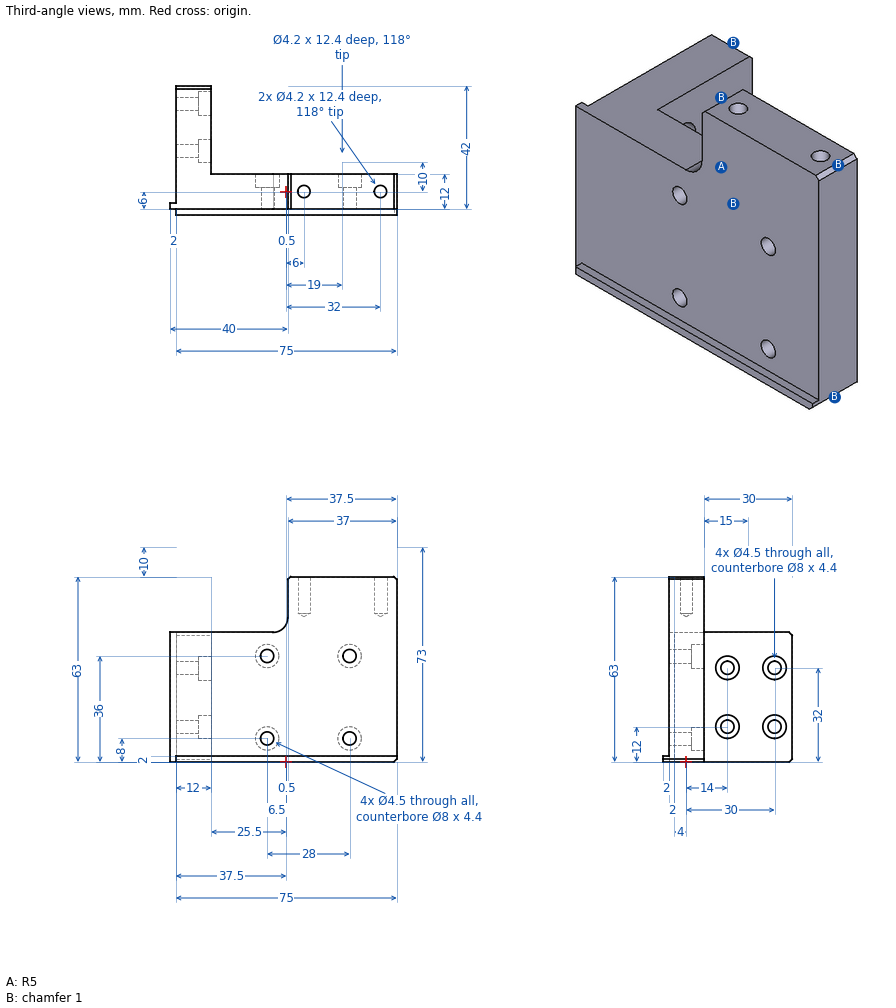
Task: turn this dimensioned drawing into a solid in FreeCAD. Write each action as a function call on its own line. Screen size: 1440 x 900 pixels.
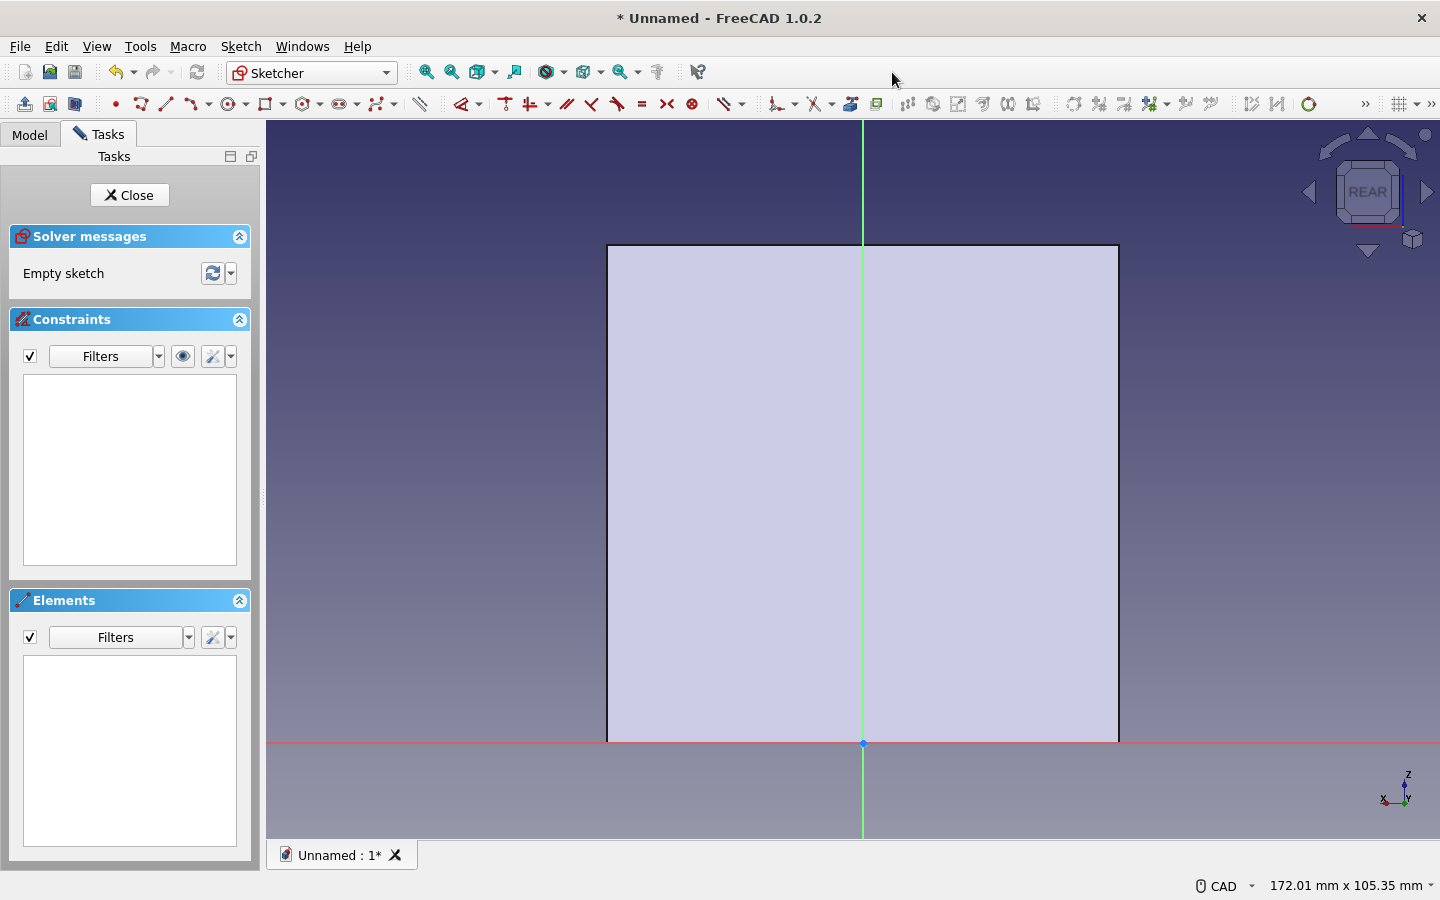
key(g)
key(r)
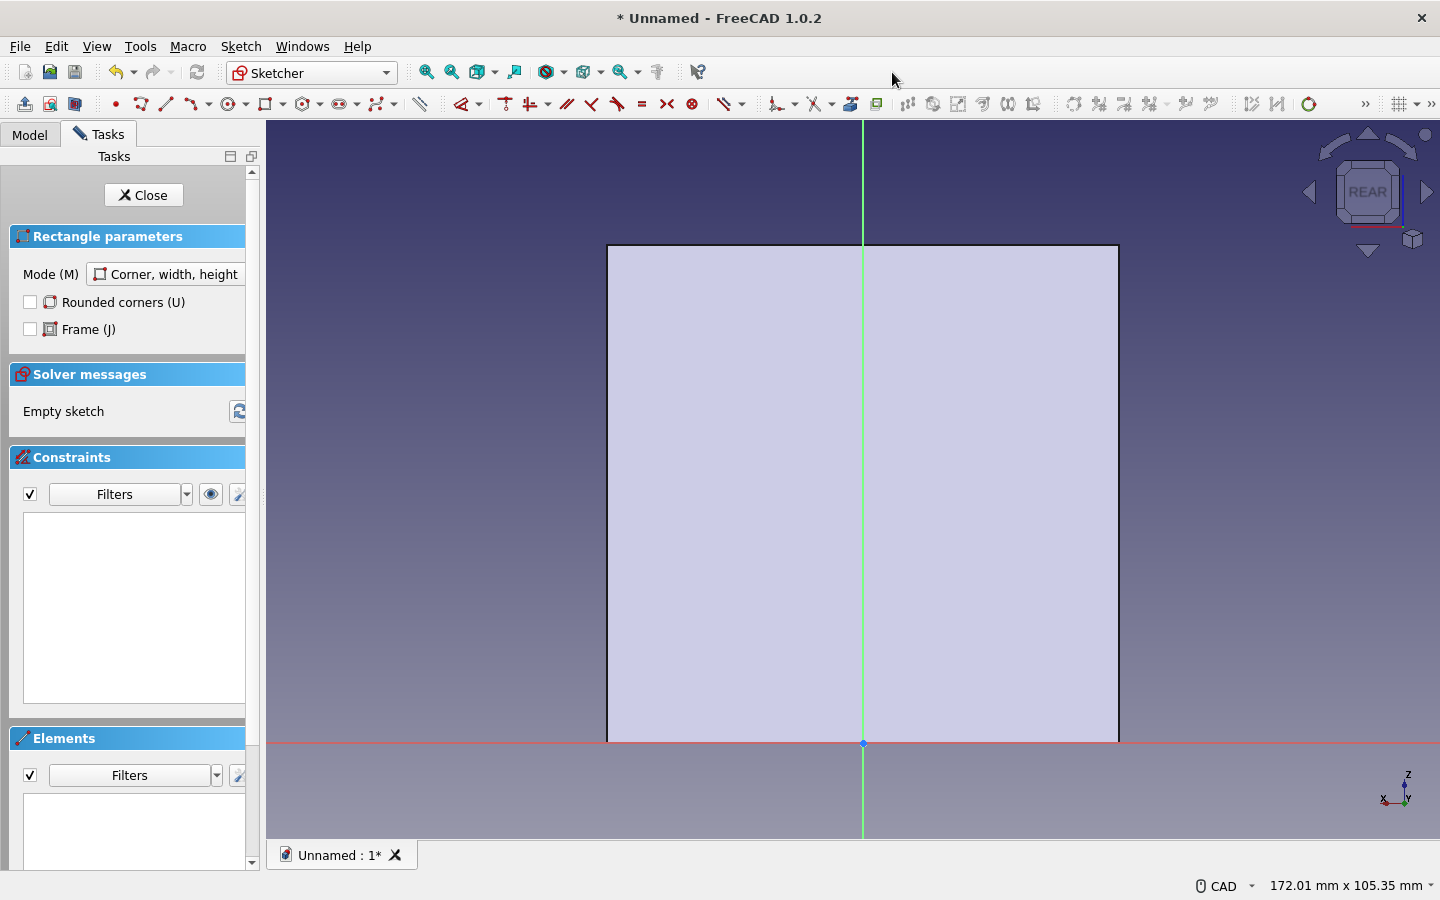
click(607, 245)
move(1119, 313)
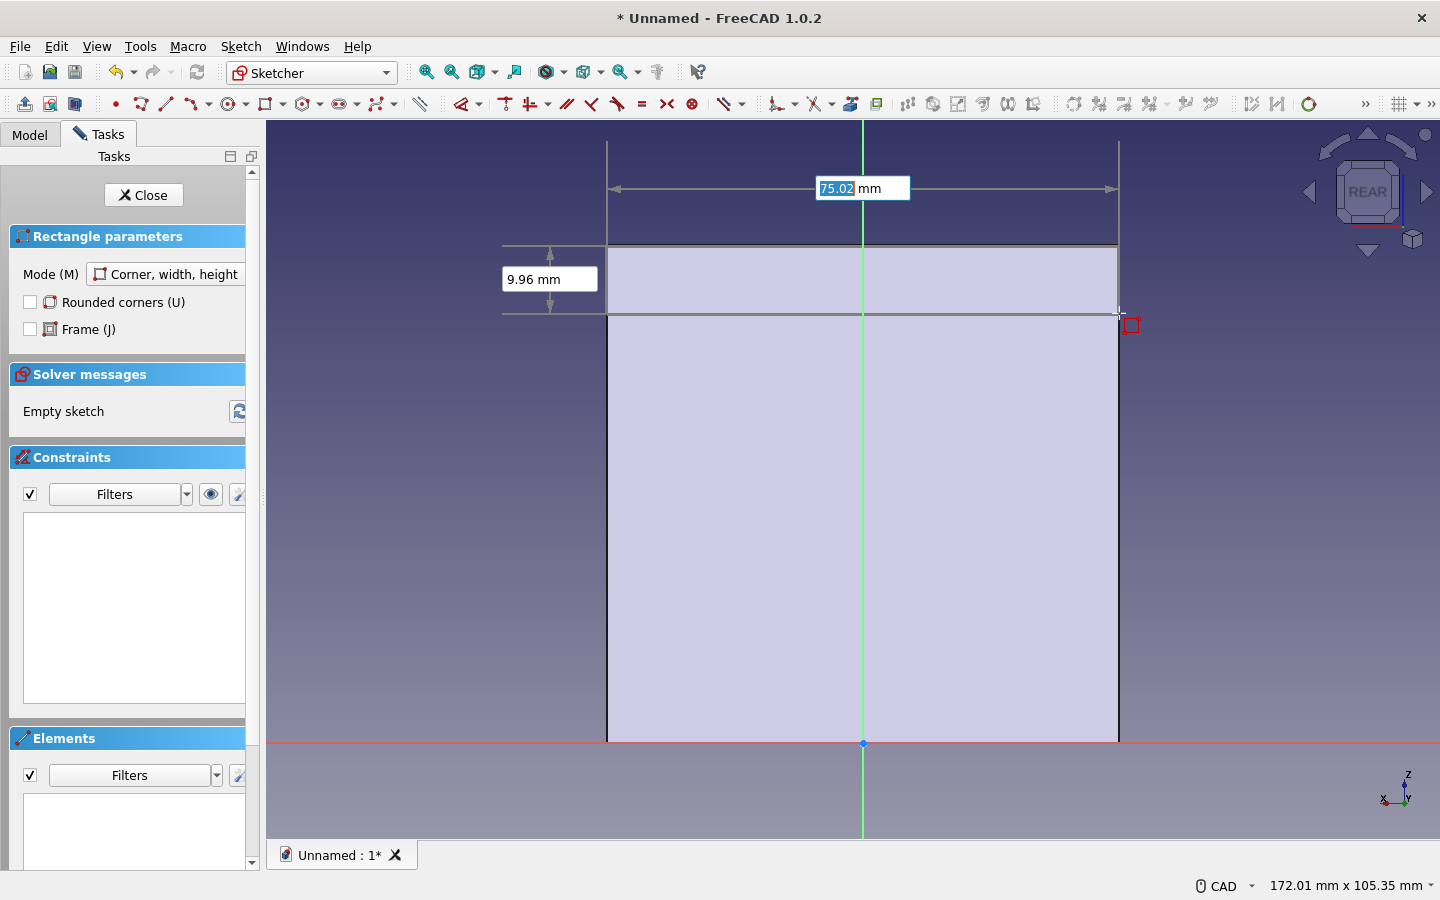
text(75)
key(Tab)
text(10)
key(Return)
key(Escape)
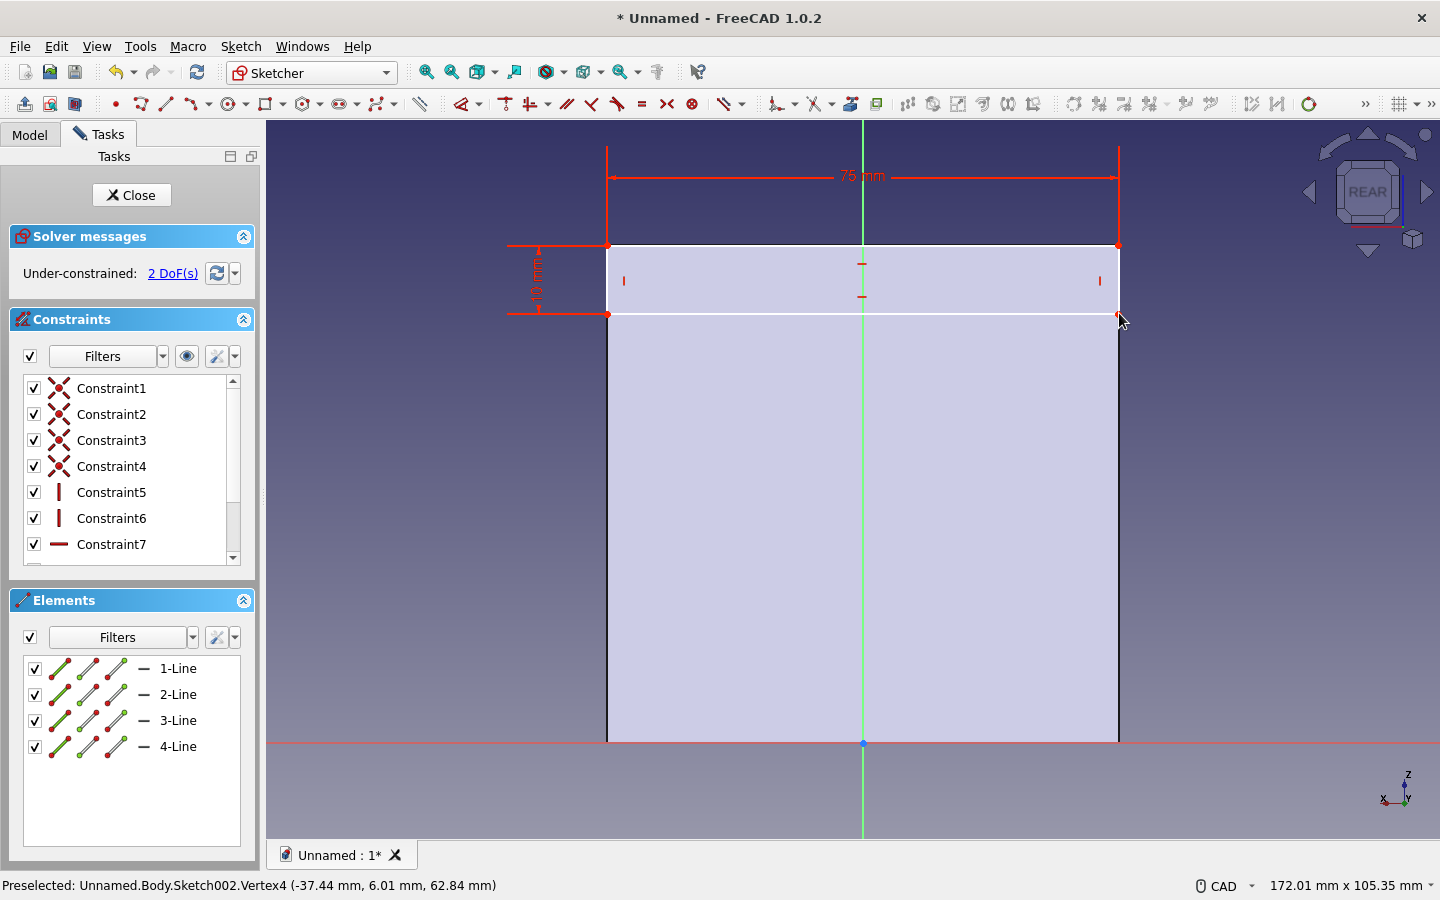
click(460, 104)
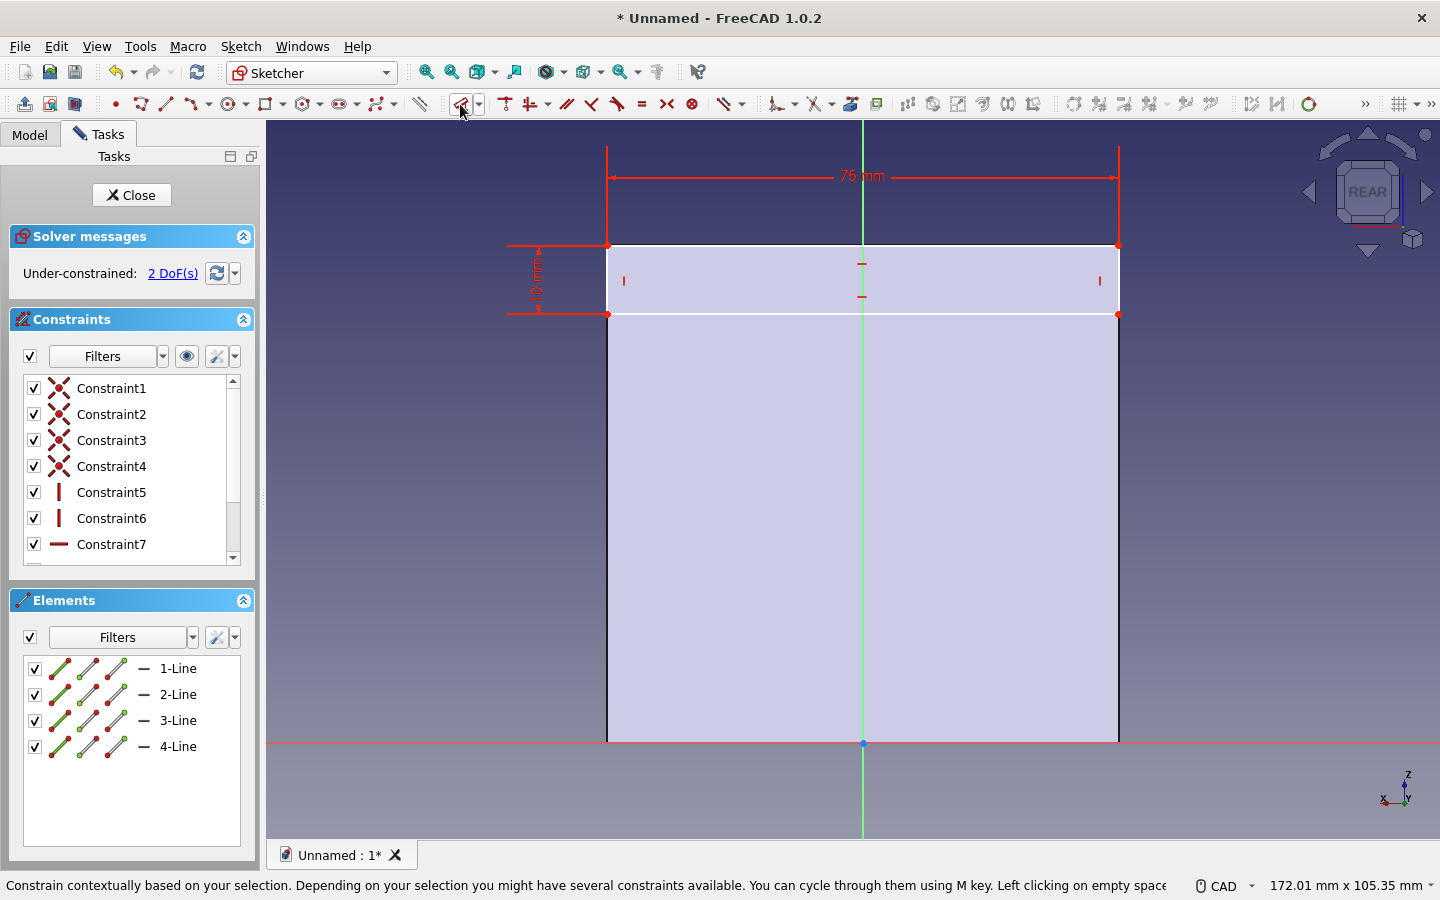
click(607, 246)
click(573, 495)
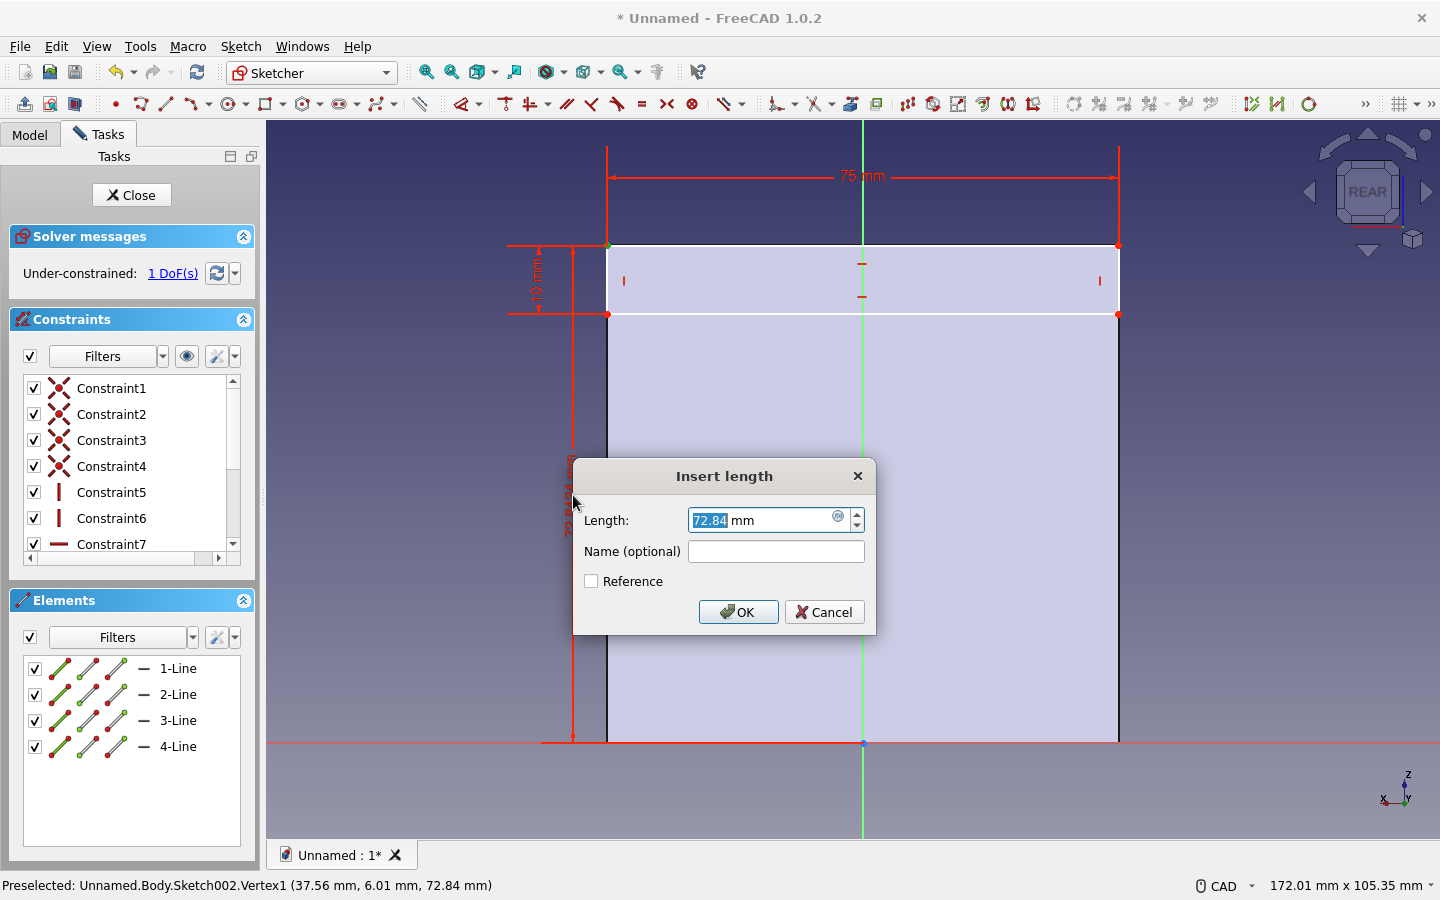
text(73)
key(Return)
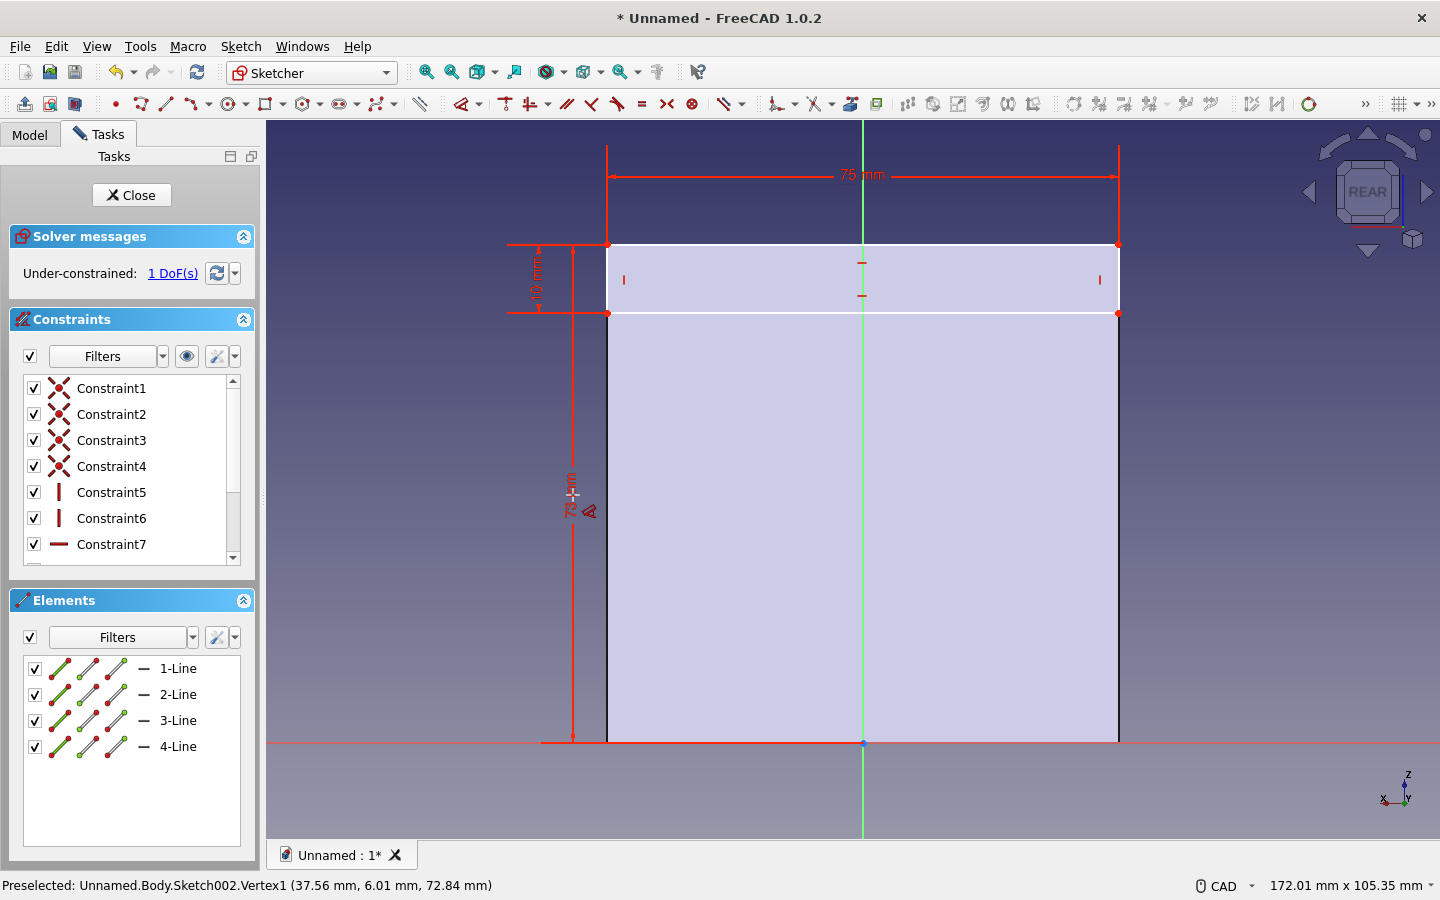
click(607, 245)
click(735, 777)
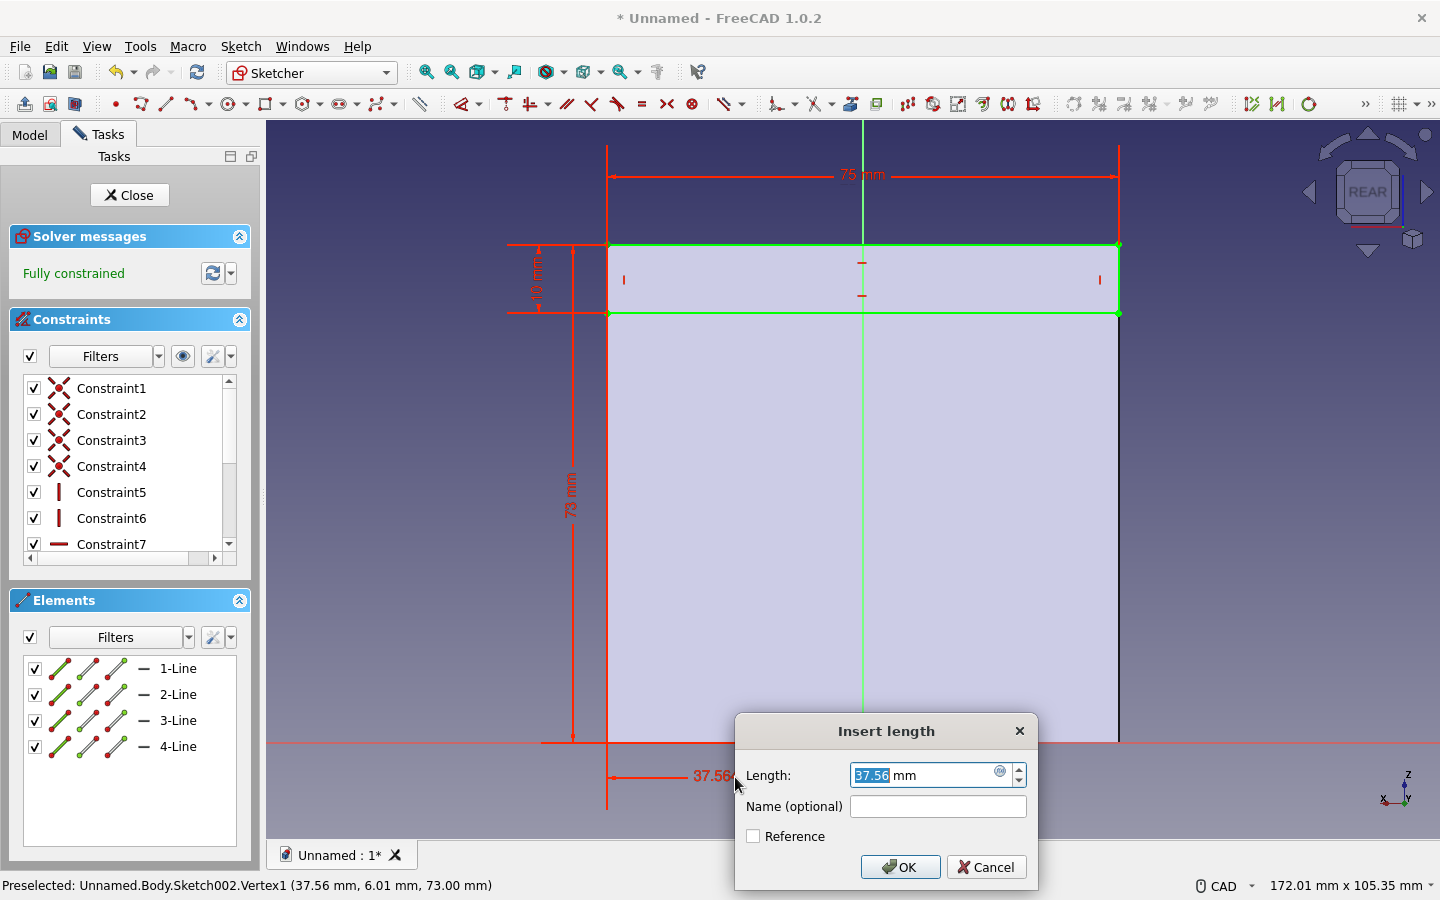
text(37.5)
key(Return)
key(Escape)